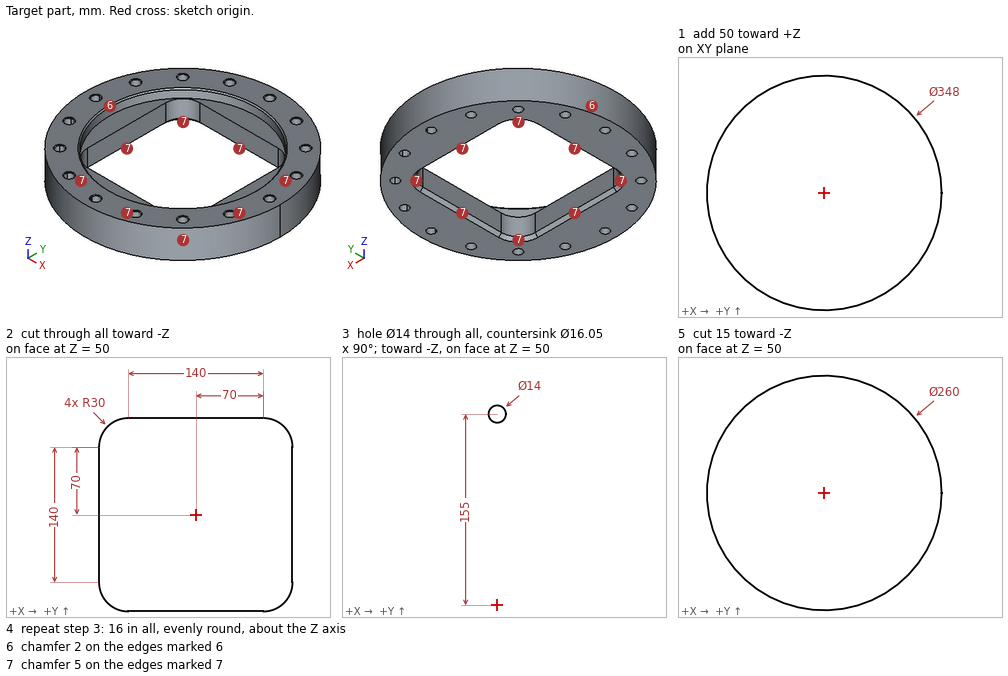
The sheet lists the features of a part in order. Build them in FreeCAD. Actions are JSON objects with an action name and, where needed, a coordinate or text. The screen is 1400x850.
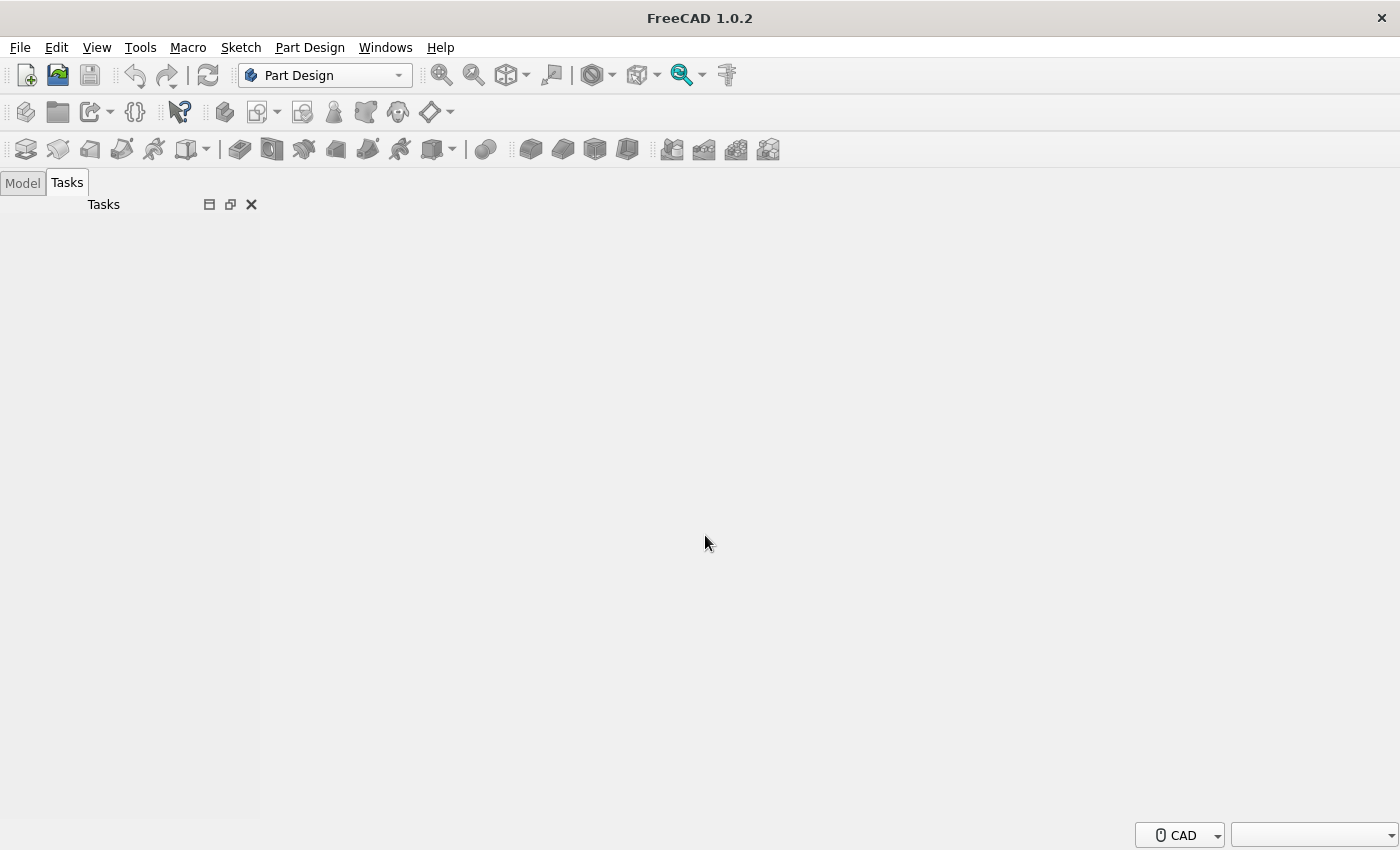
{"action": "left_click", "coordinate": [26, 76]}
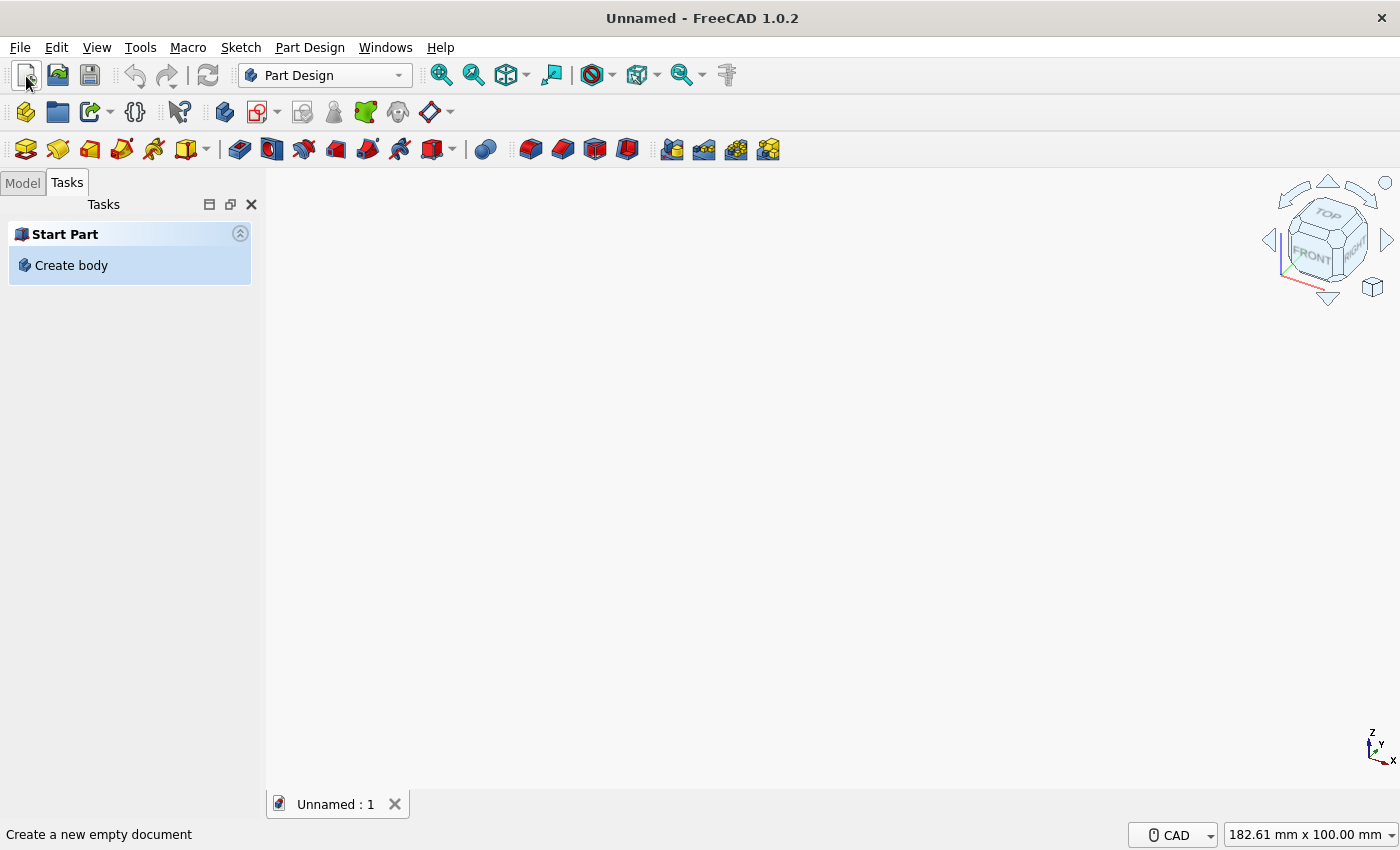
{"action": "left_click", "coordinate": [258, 112]}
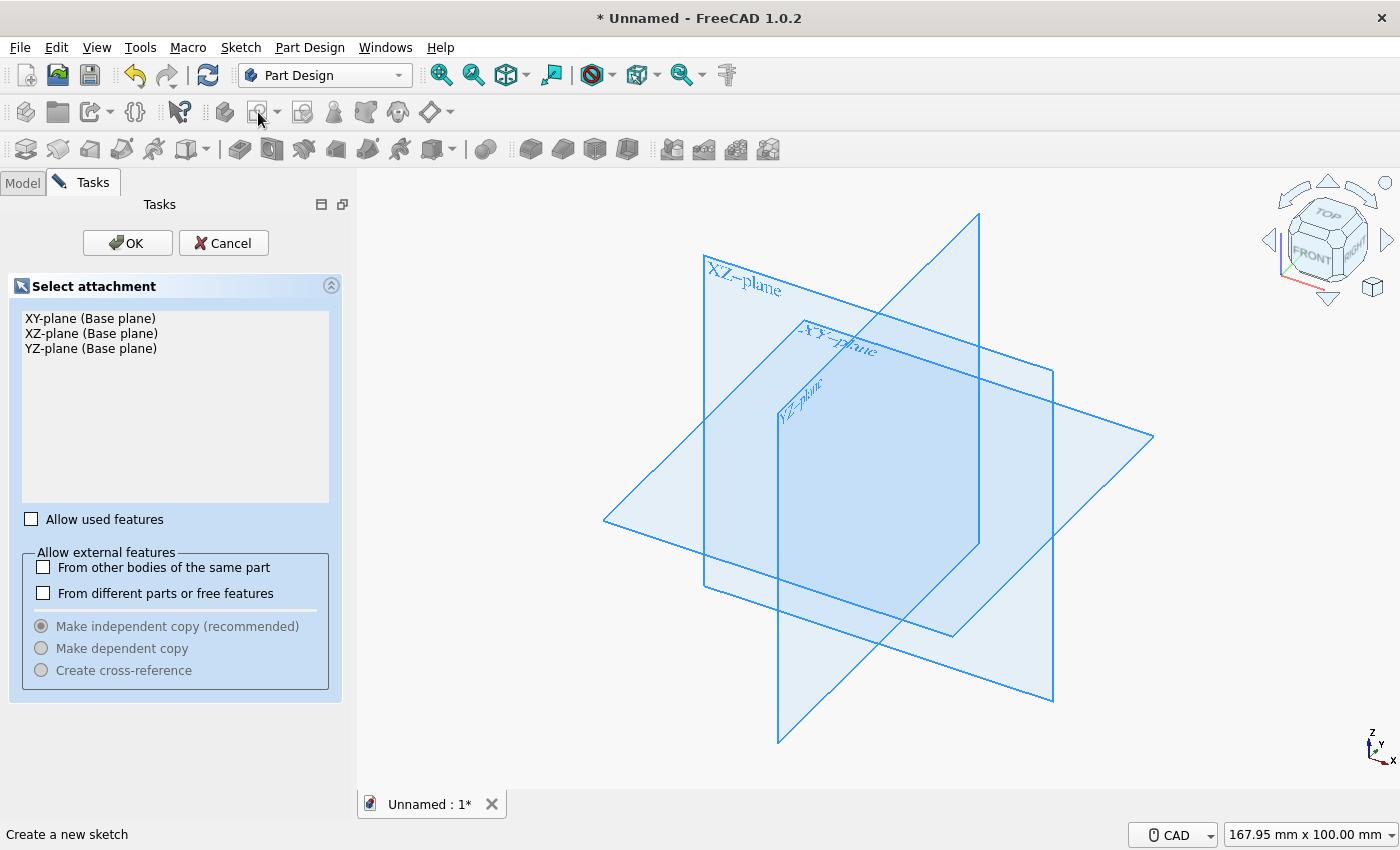
{"action": "left_click", "coordinate": [82, 318]}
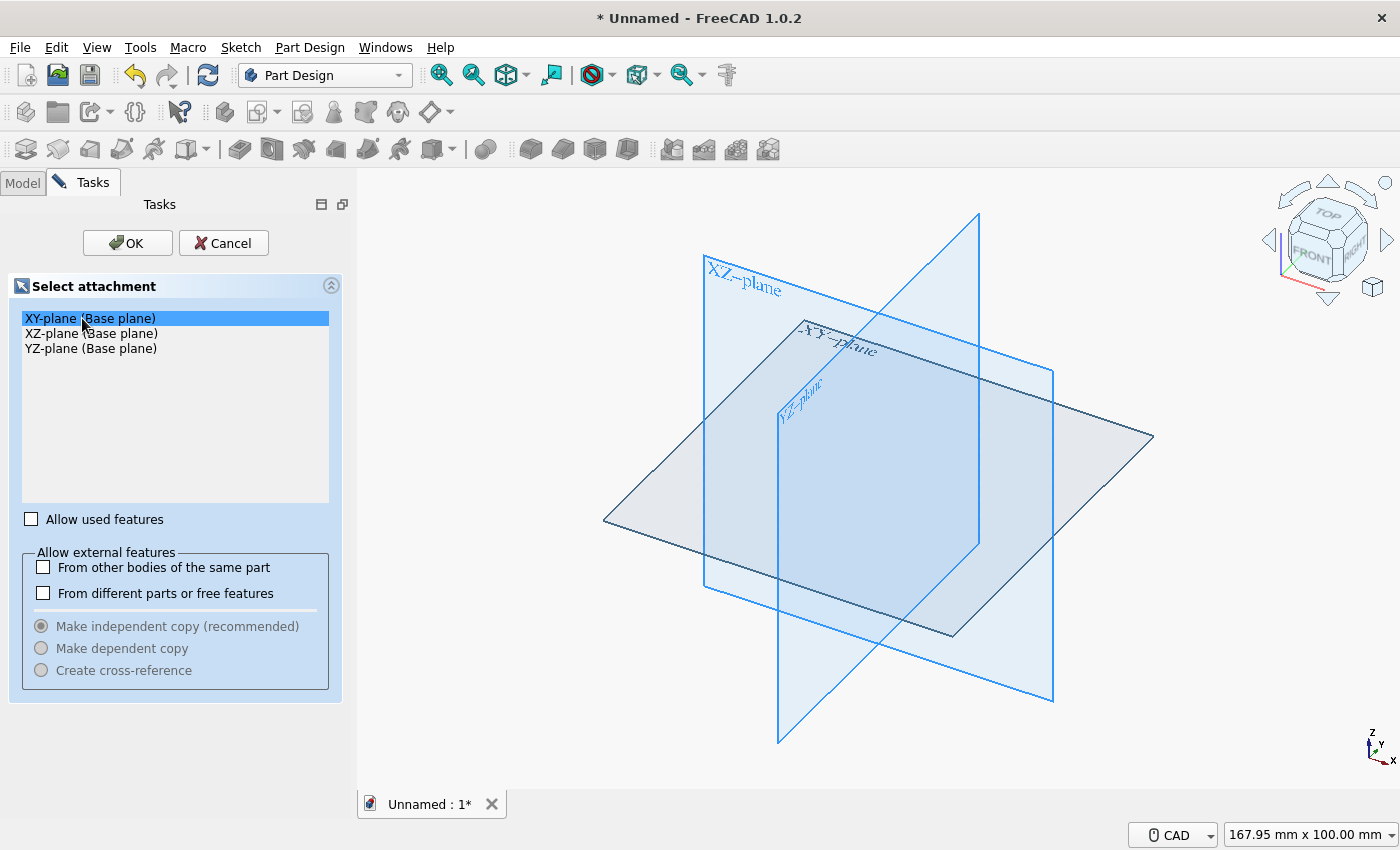
{"action": "left_click", "coordinate": [128, 243]}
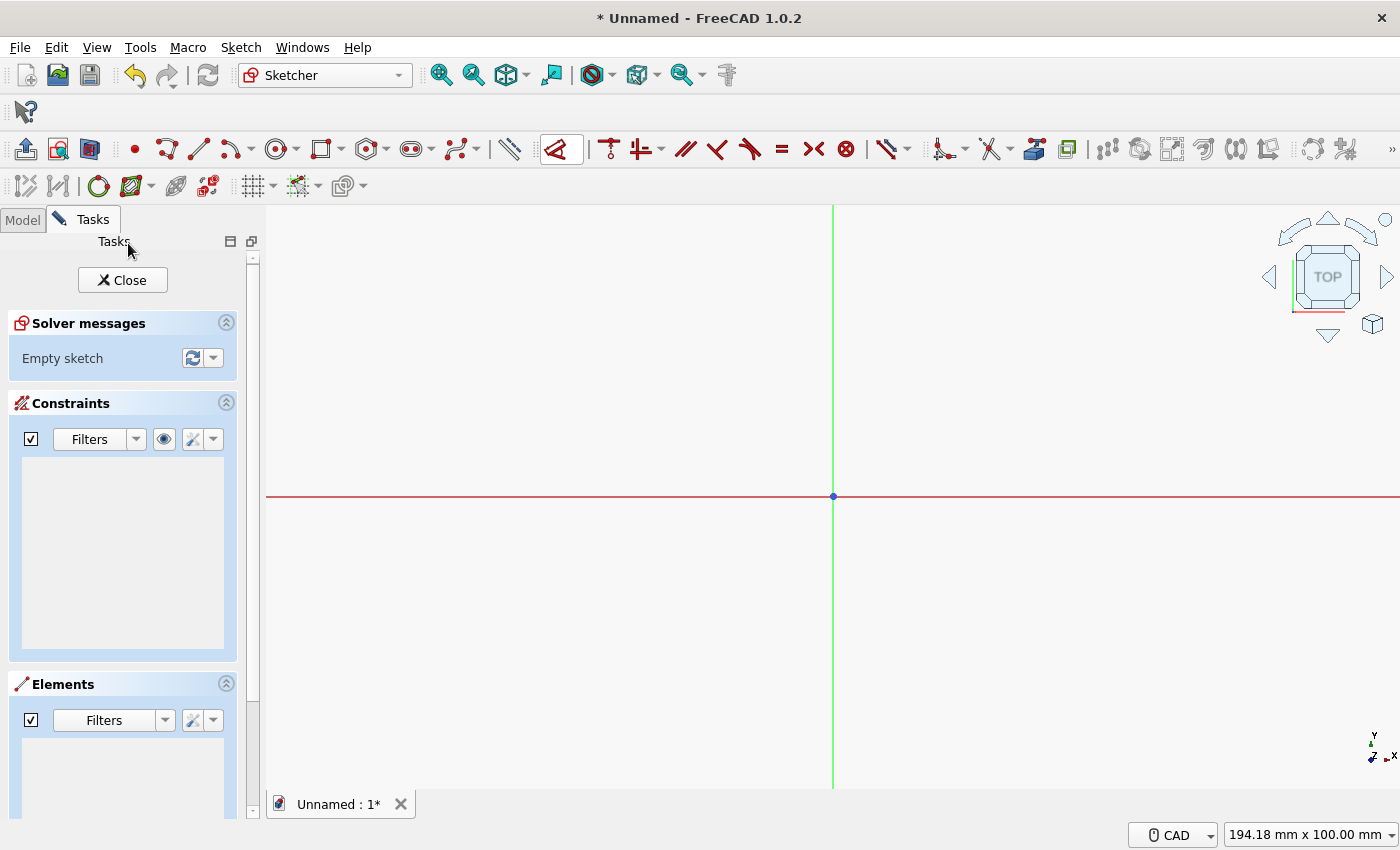
{"action": "scroll", "coordinate": [747, 497], "scroll_direction": "down", "scroll_amount": 8}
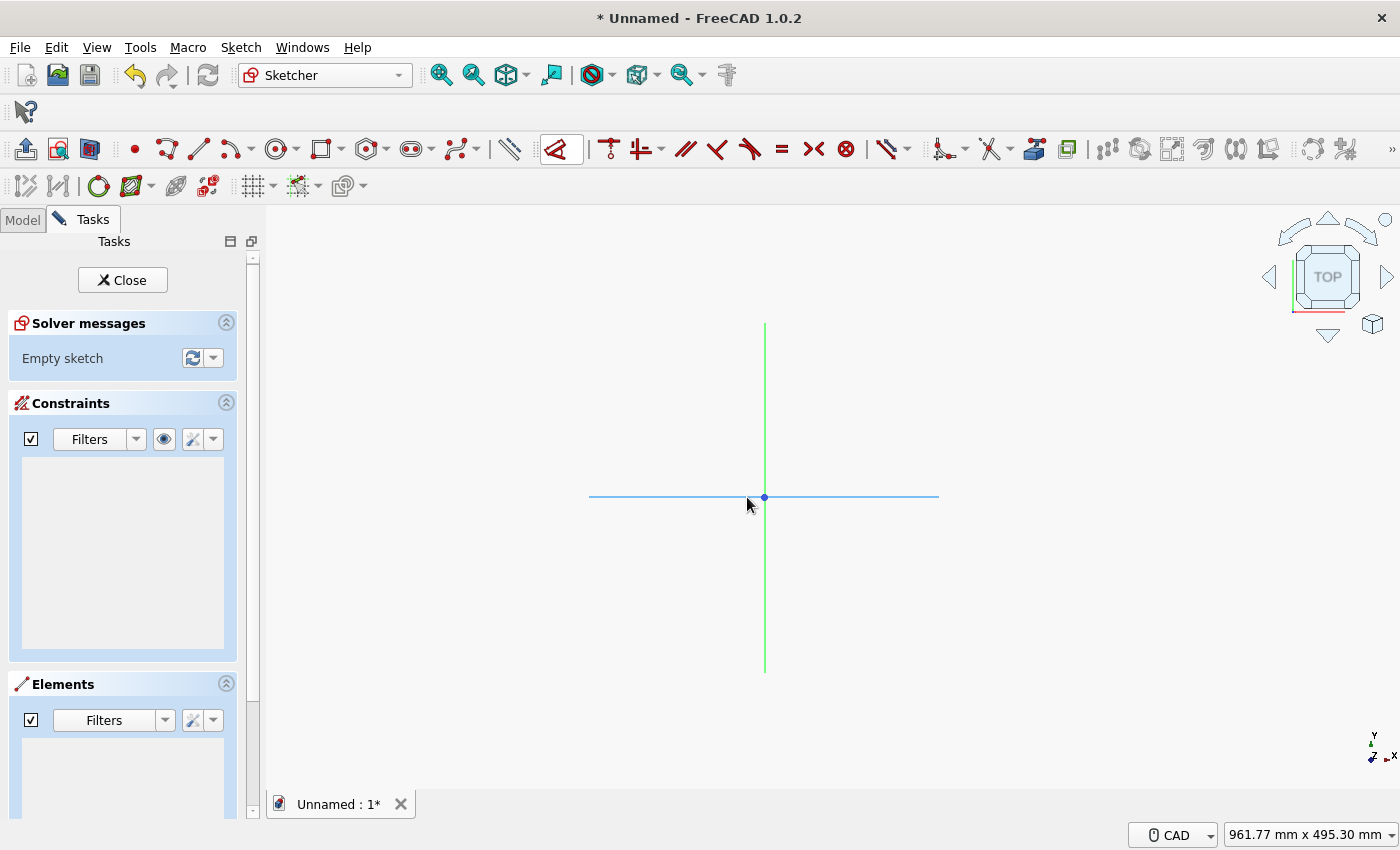
{"action": "left_click", "coordinate": [276, 150]}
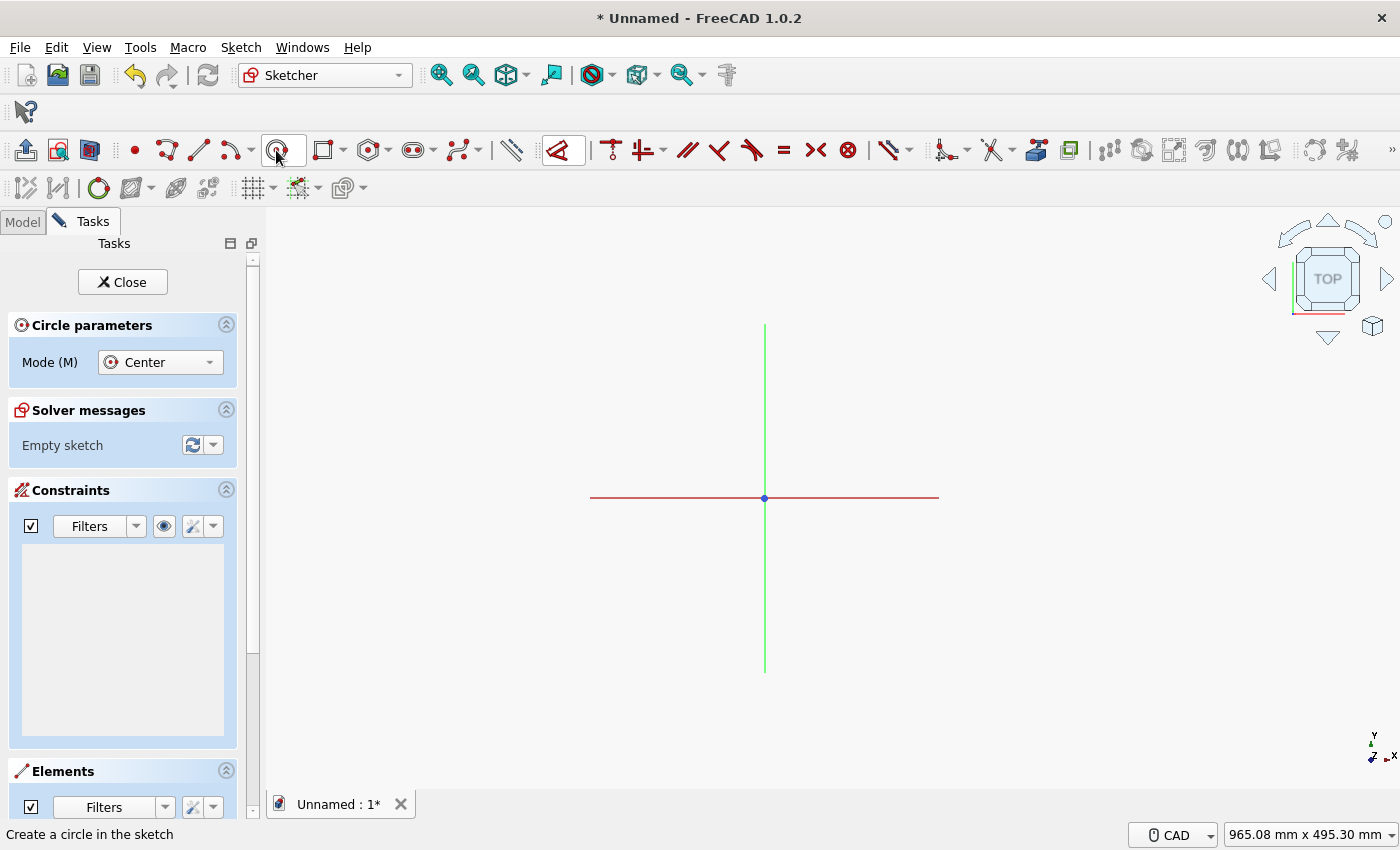
{"action": "left_click", "coordinate": [765, 498]}
{"action": "left_click", "coordinate": [910, 354]}
{"action": "key", "text": "Escape"}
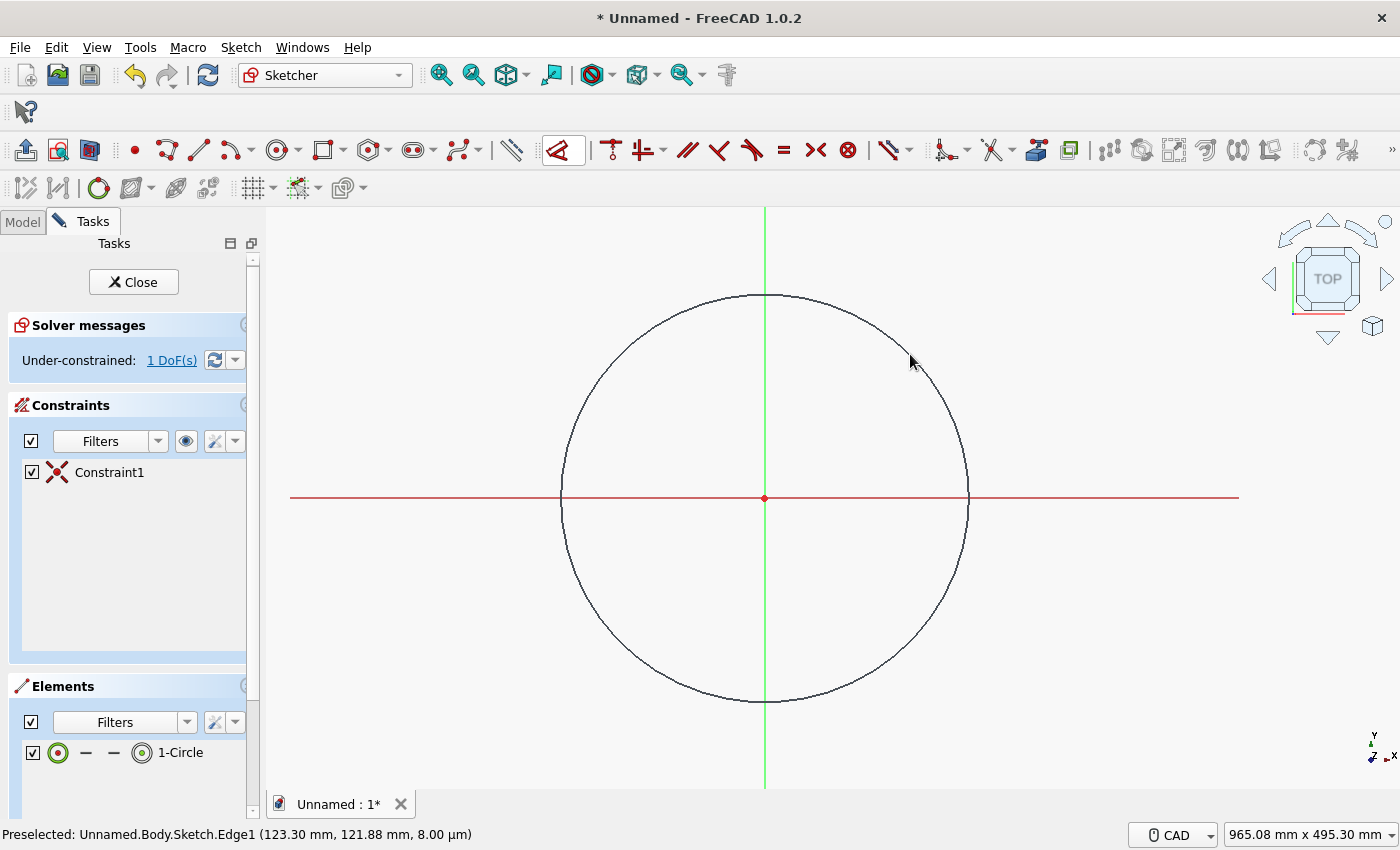
{"action": "left_click", "coordinate": [558, 150]}